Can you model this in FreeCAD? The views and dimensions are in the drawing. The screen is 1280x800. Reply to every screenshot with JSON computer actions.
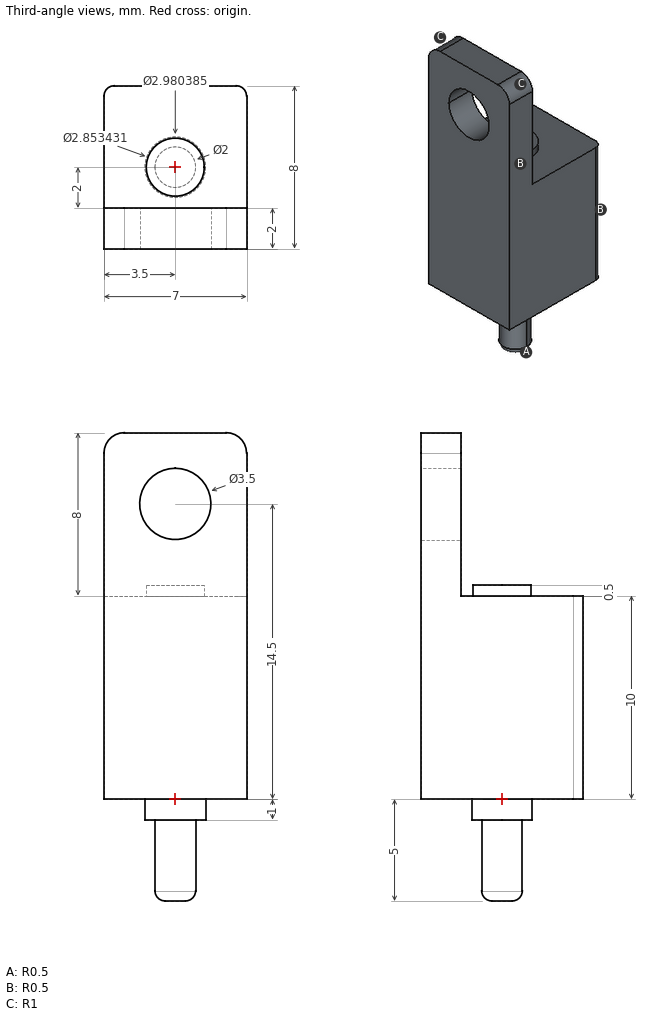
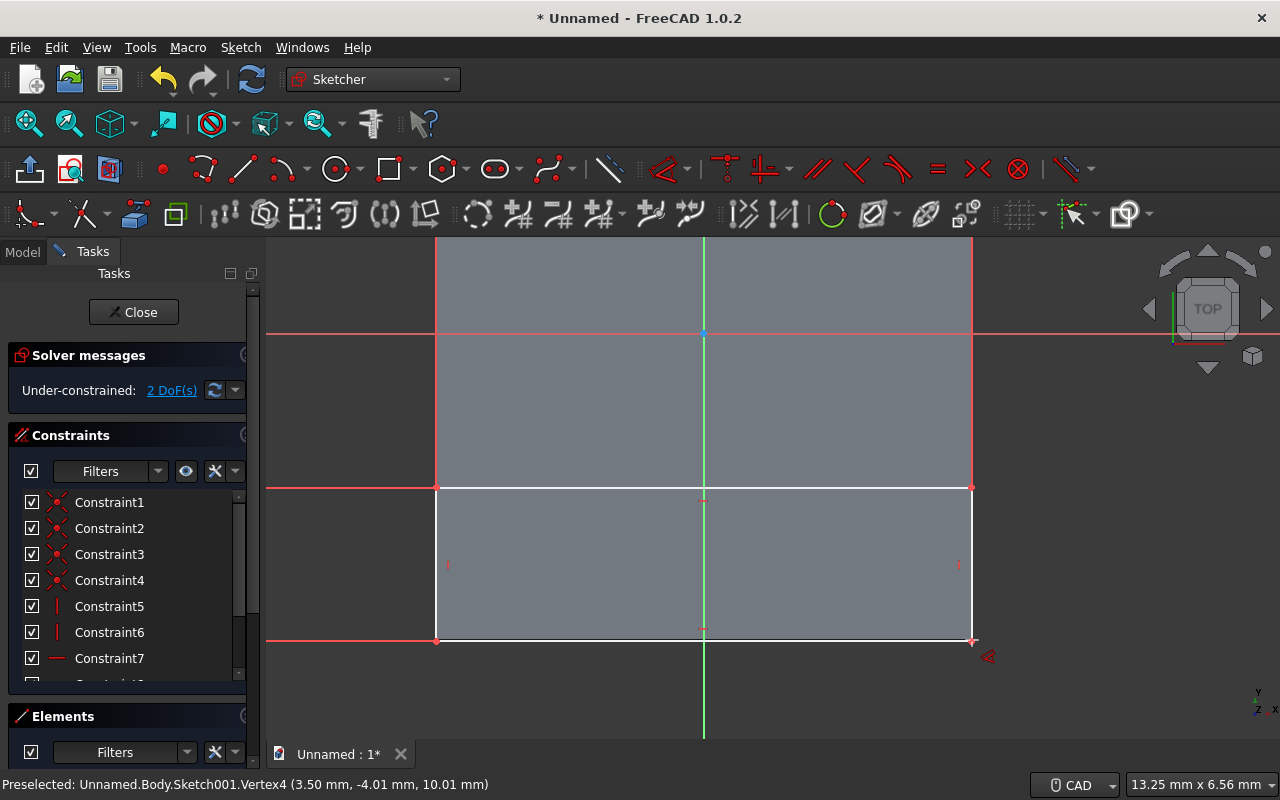
{"action": "left_click", "coordinate": [436, 488]}
{"action": "left_click", "coordinate": [402, 411]}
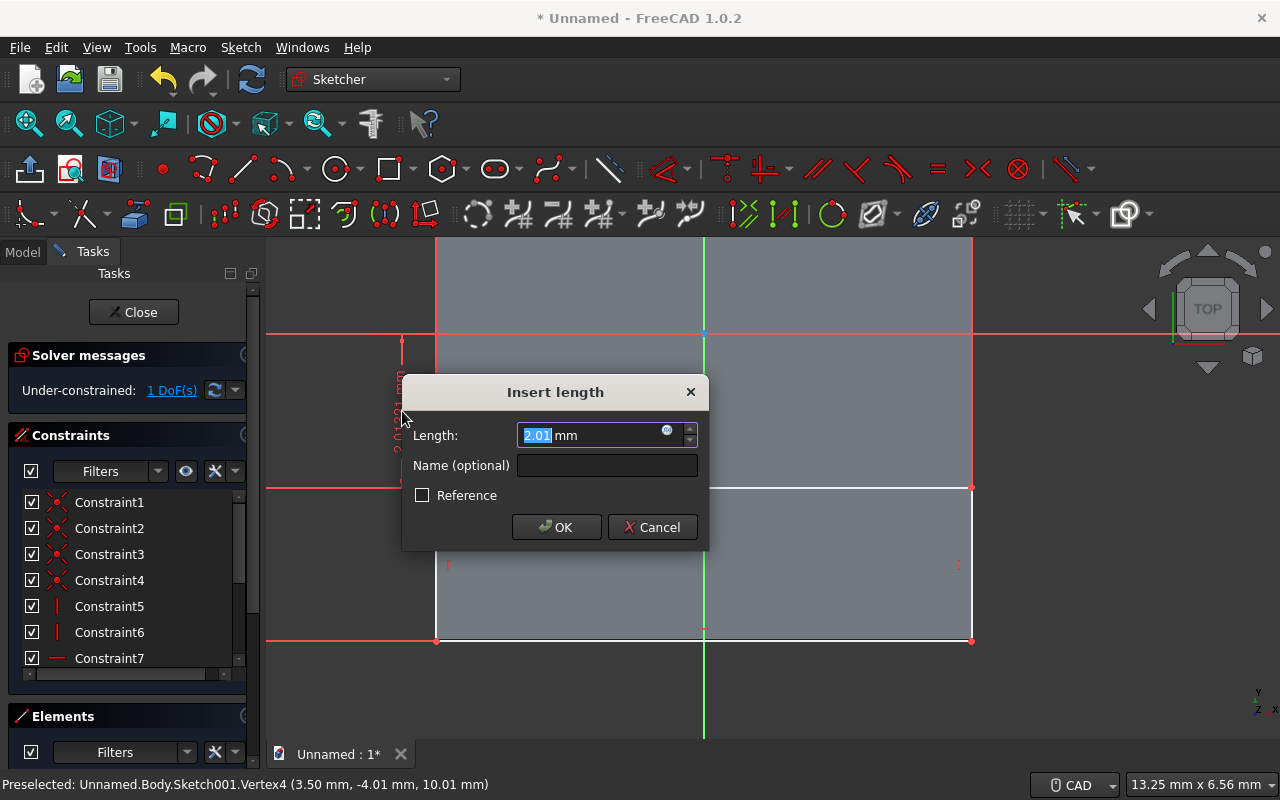
{"action": "type", "text": "2"}
{"action": "key", "text": "Return"}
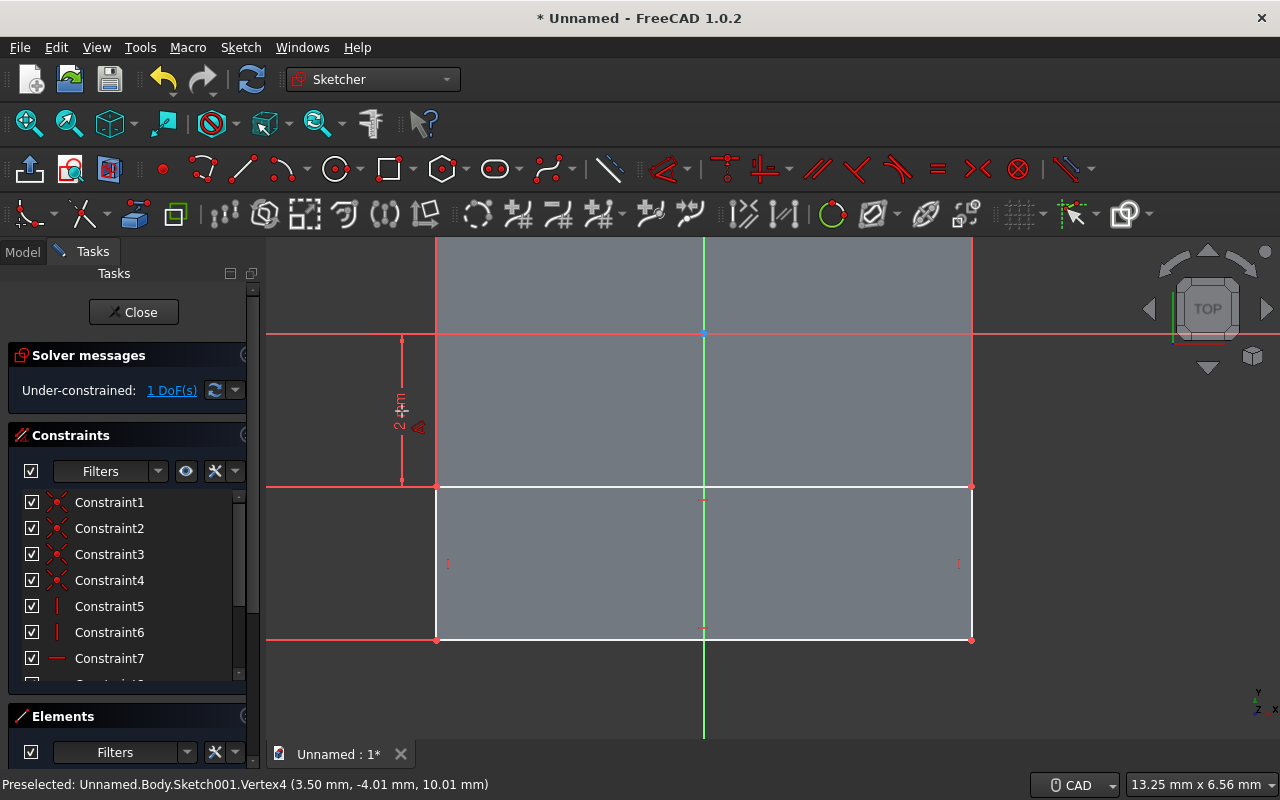
{"action": "left_click", "coordinate": [436, 487]}
{"action": "left_click", "coordinate": [570, 300]}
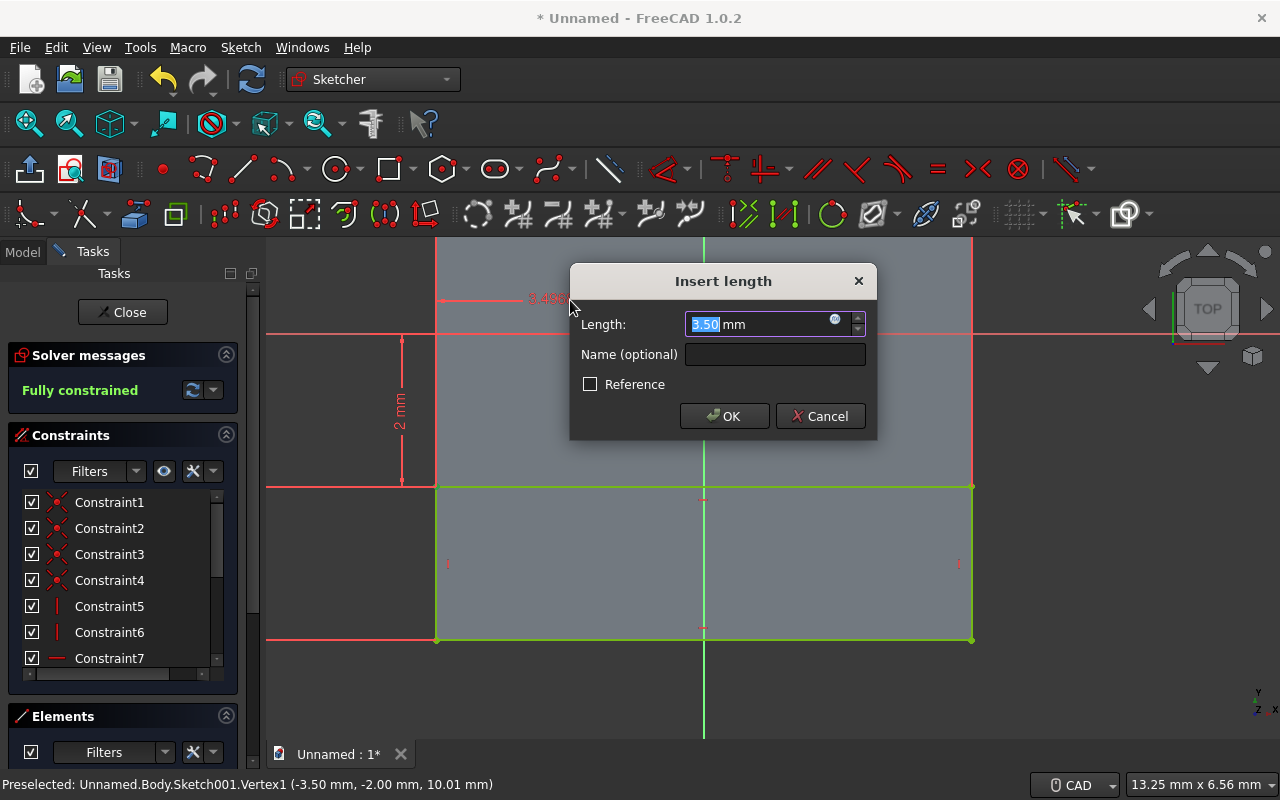
{"action": "type", "text": "3.5"}
{"action": "key", "text": "Return"}
{"action": "key", "text": "Escape"}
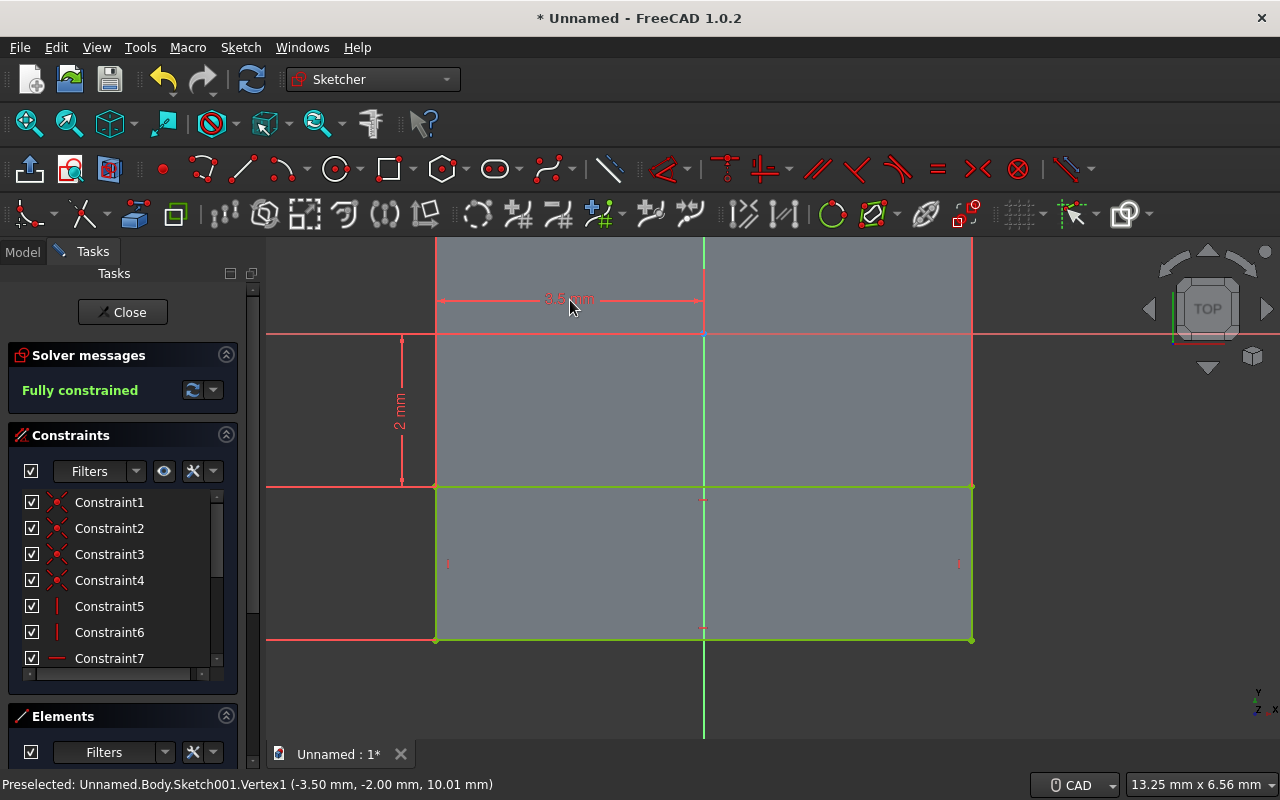
{"action": "left_click", "coordinate": [123, 312]}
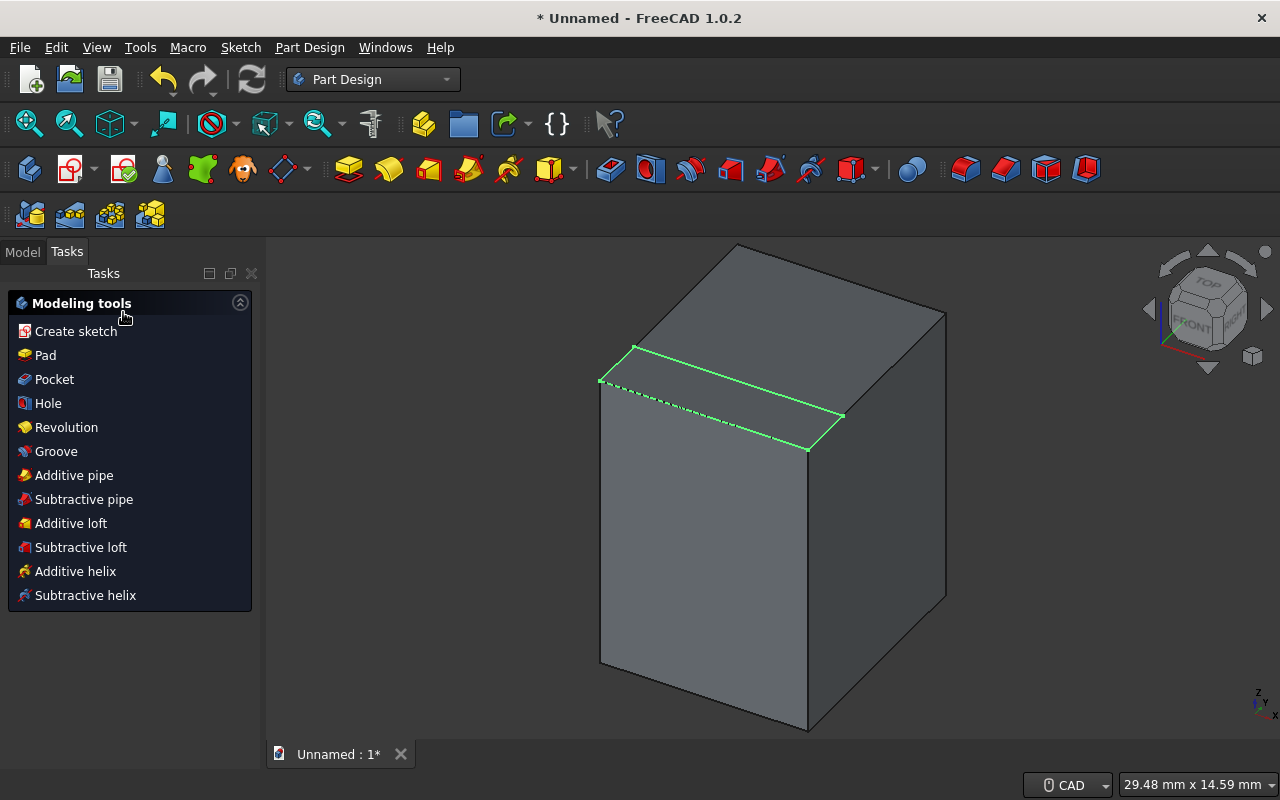
{"action": "left_click", "coordinate": [350, 170]}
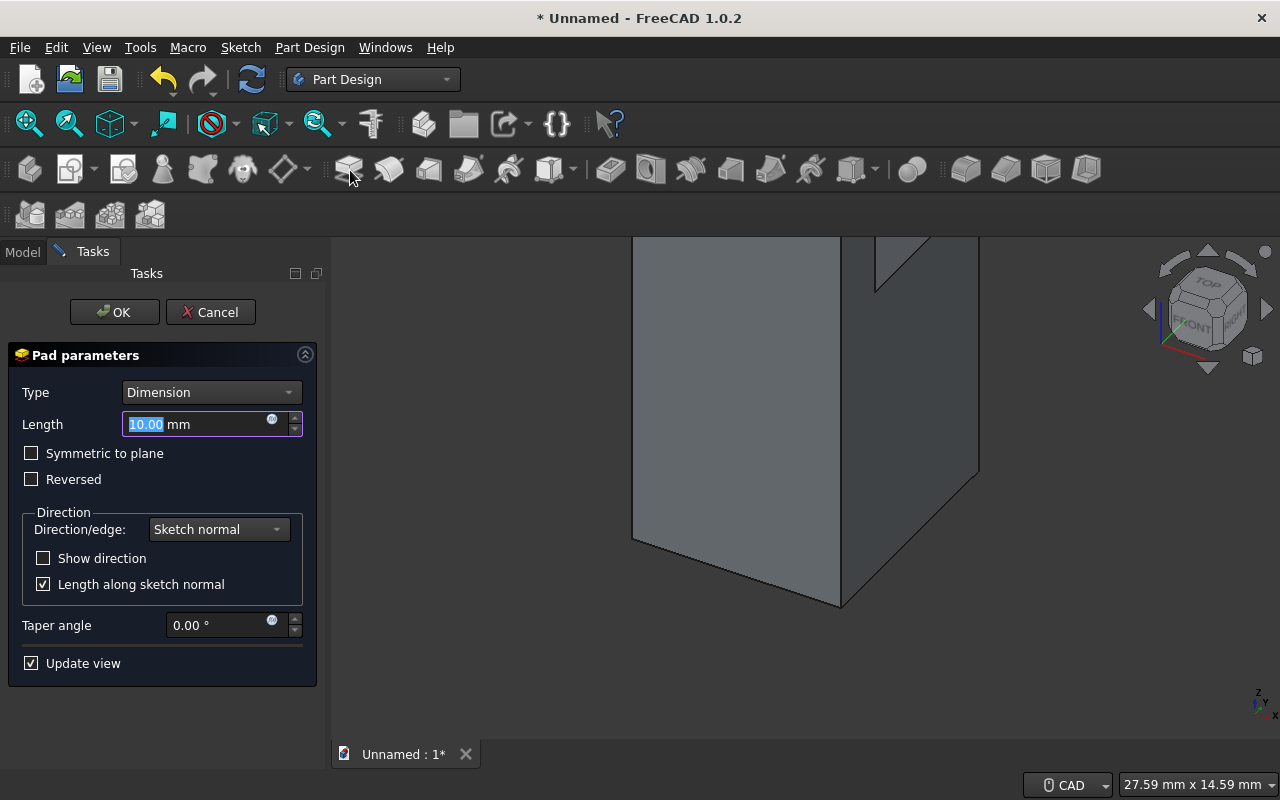
{"action": "type", "text": "8"}
{"action": "key", "text": "Tab"}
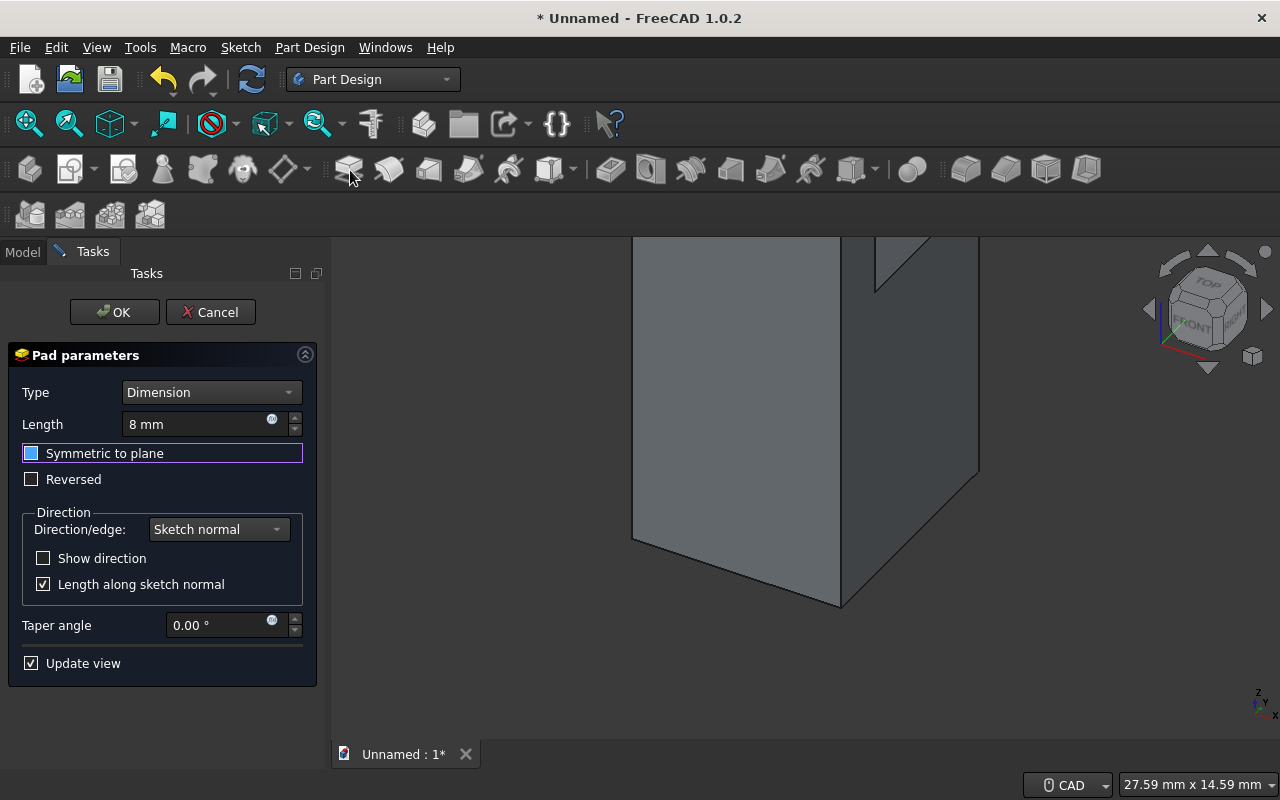
{"action": "left_click", "coordinate": [115, 312]}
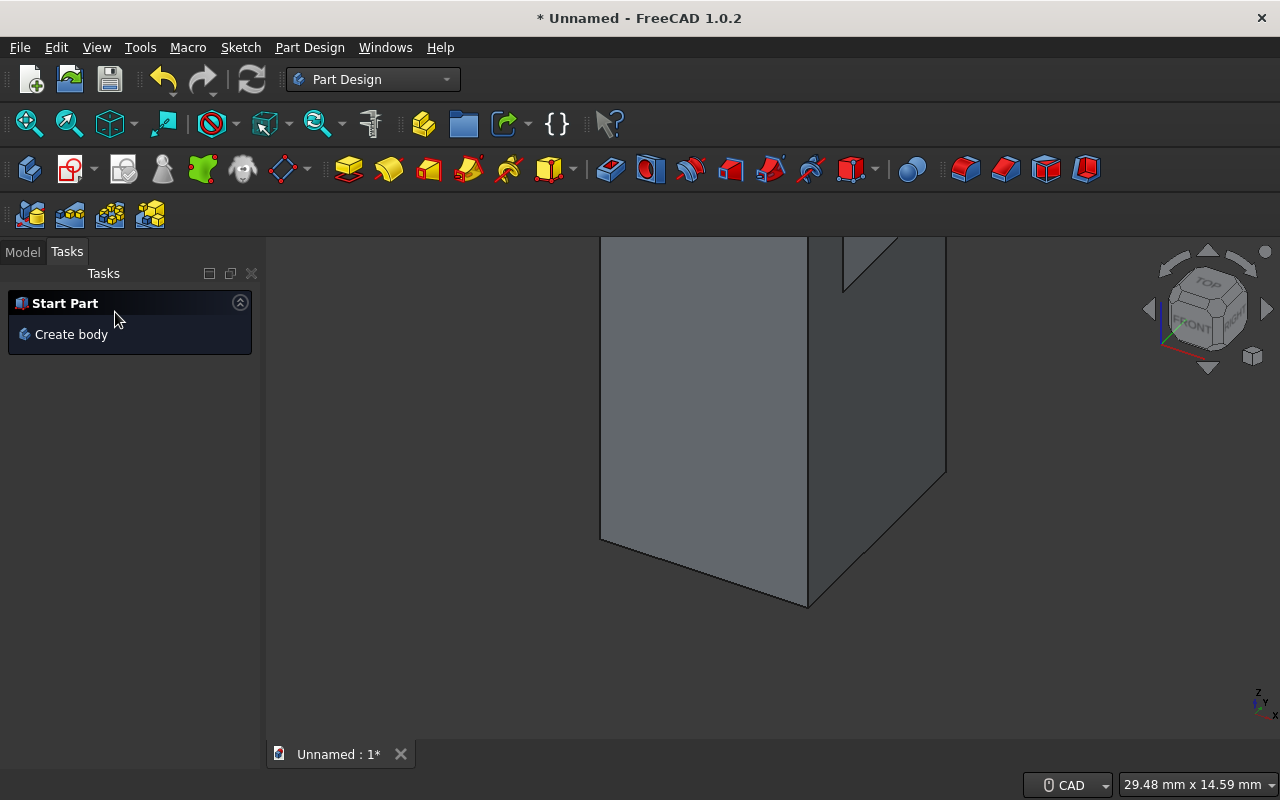
{"action": "key", "text": "v f"}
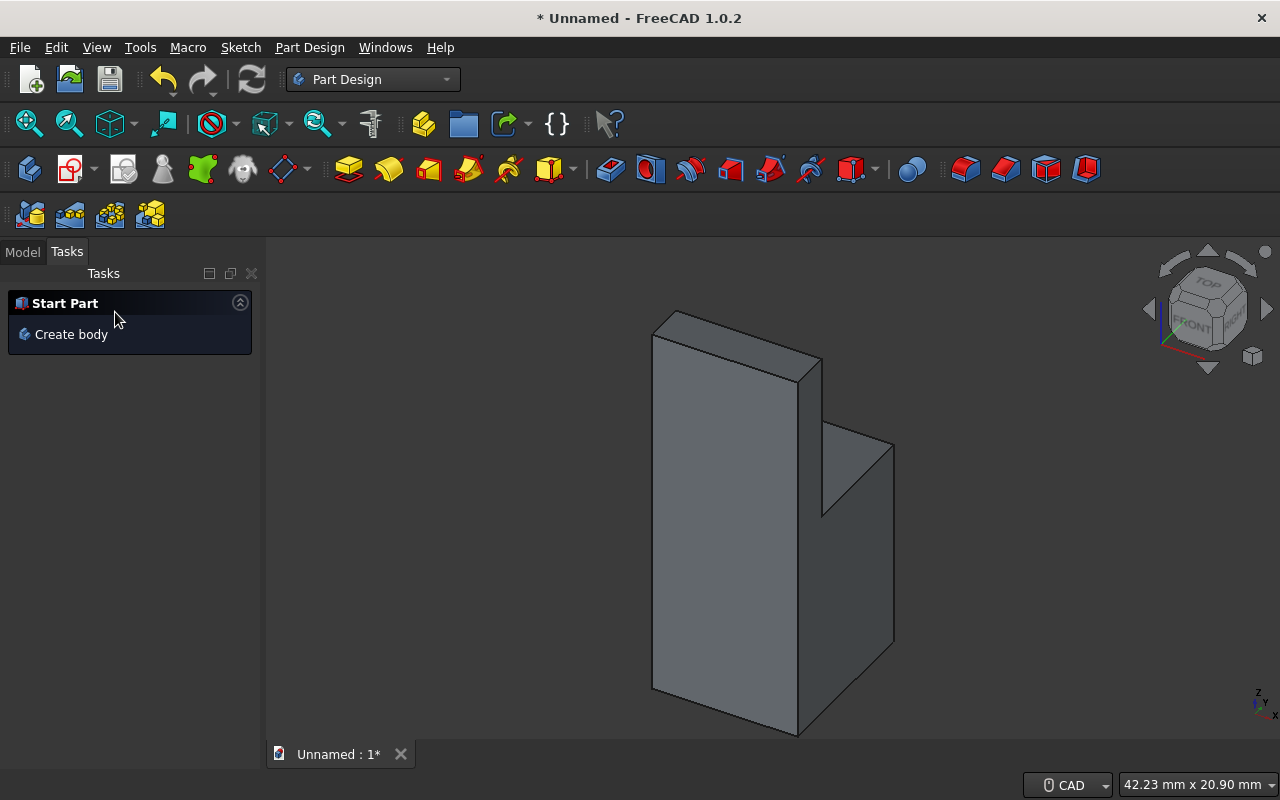
{"action": "key", "text": "5"}